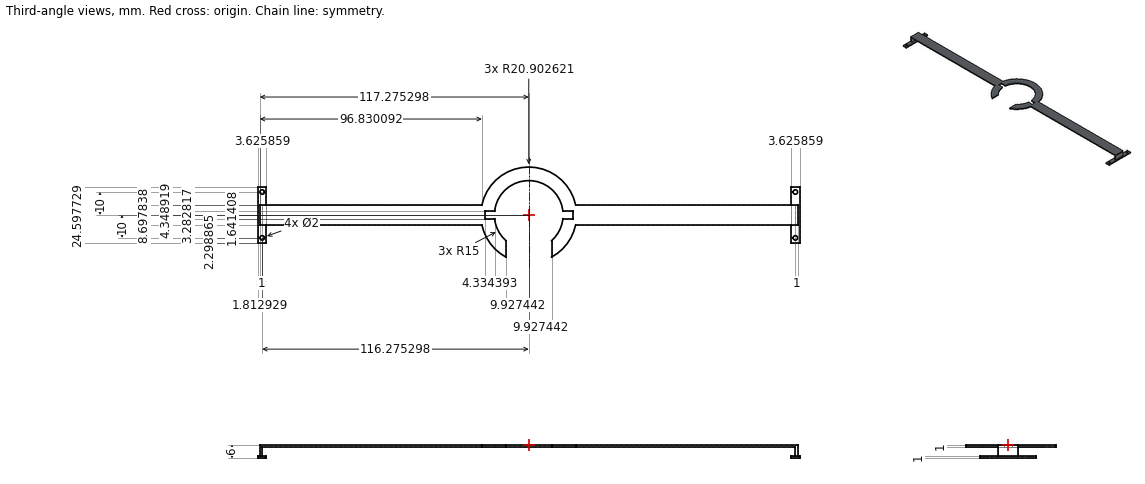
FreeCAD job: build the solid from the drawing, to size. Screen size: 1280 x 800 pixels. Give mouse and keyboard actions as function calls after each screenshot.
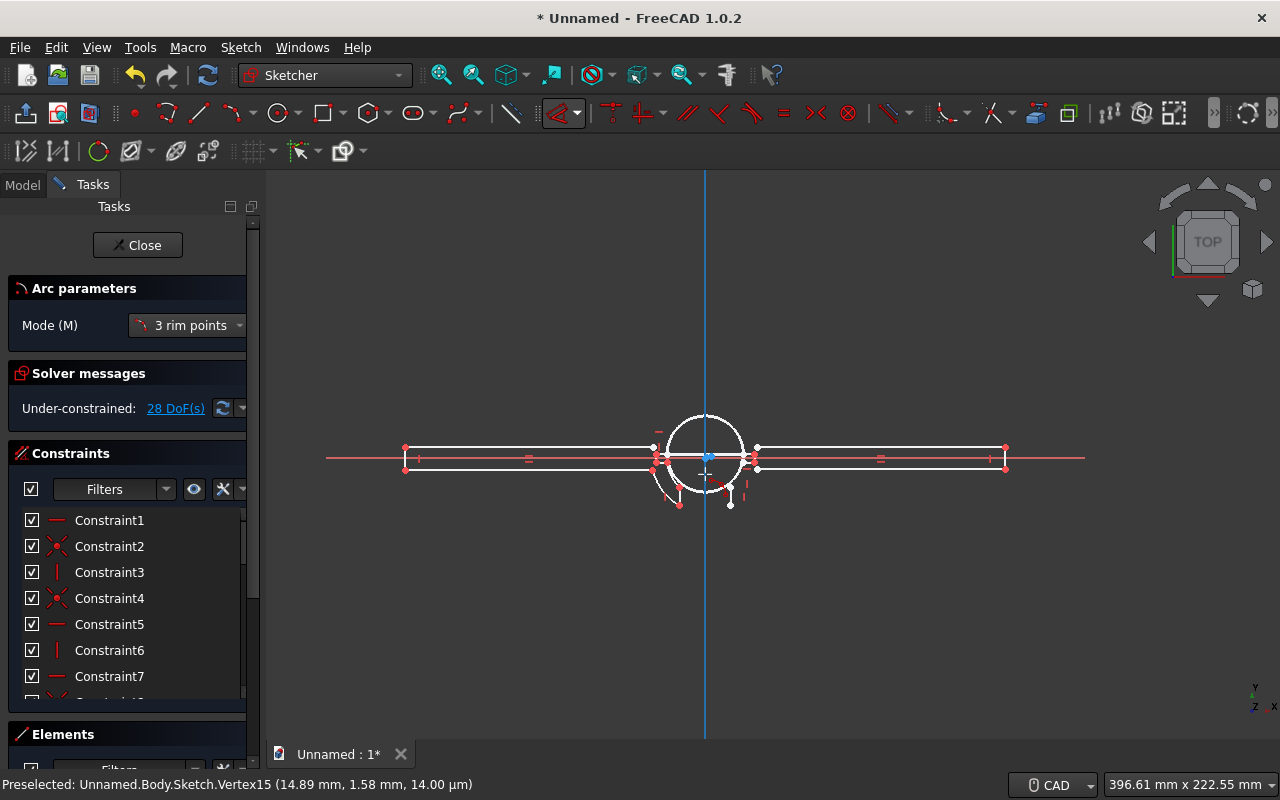
click(726, 426)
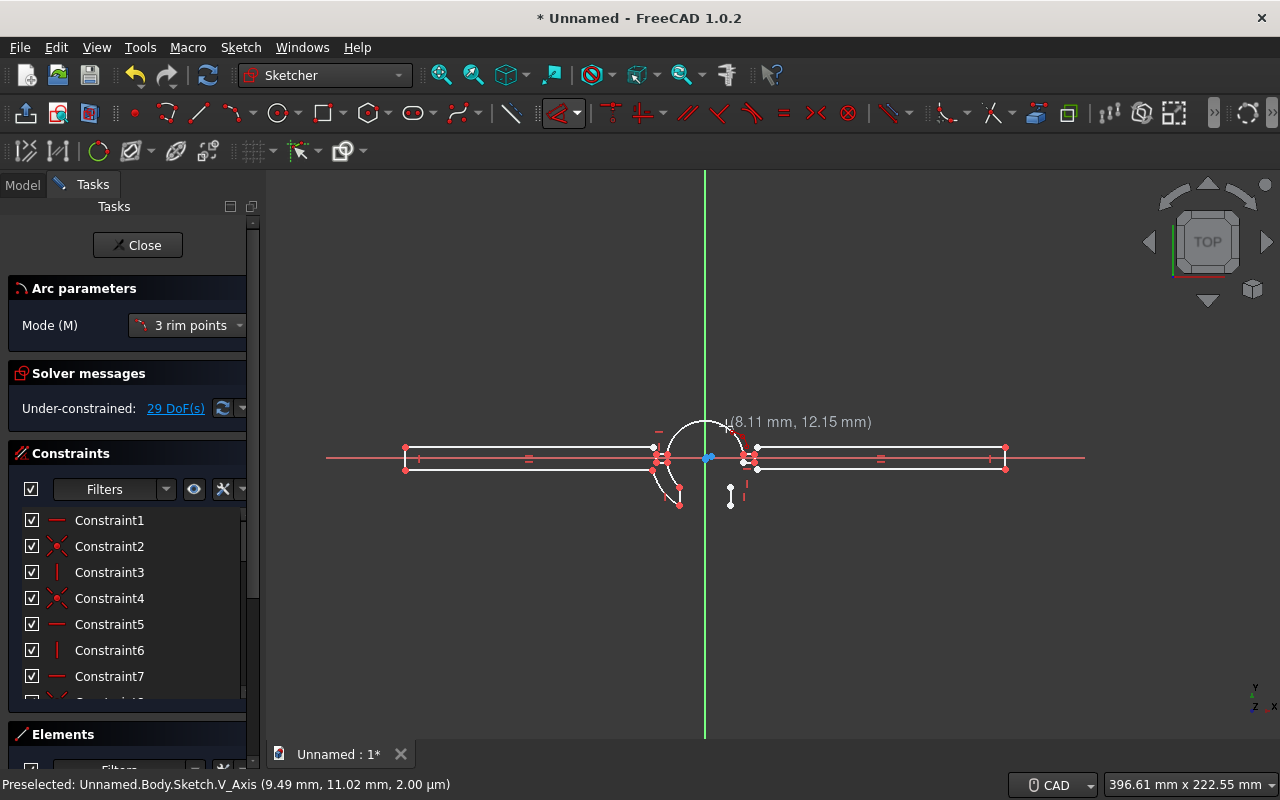
scroll(743, 462, up, 7)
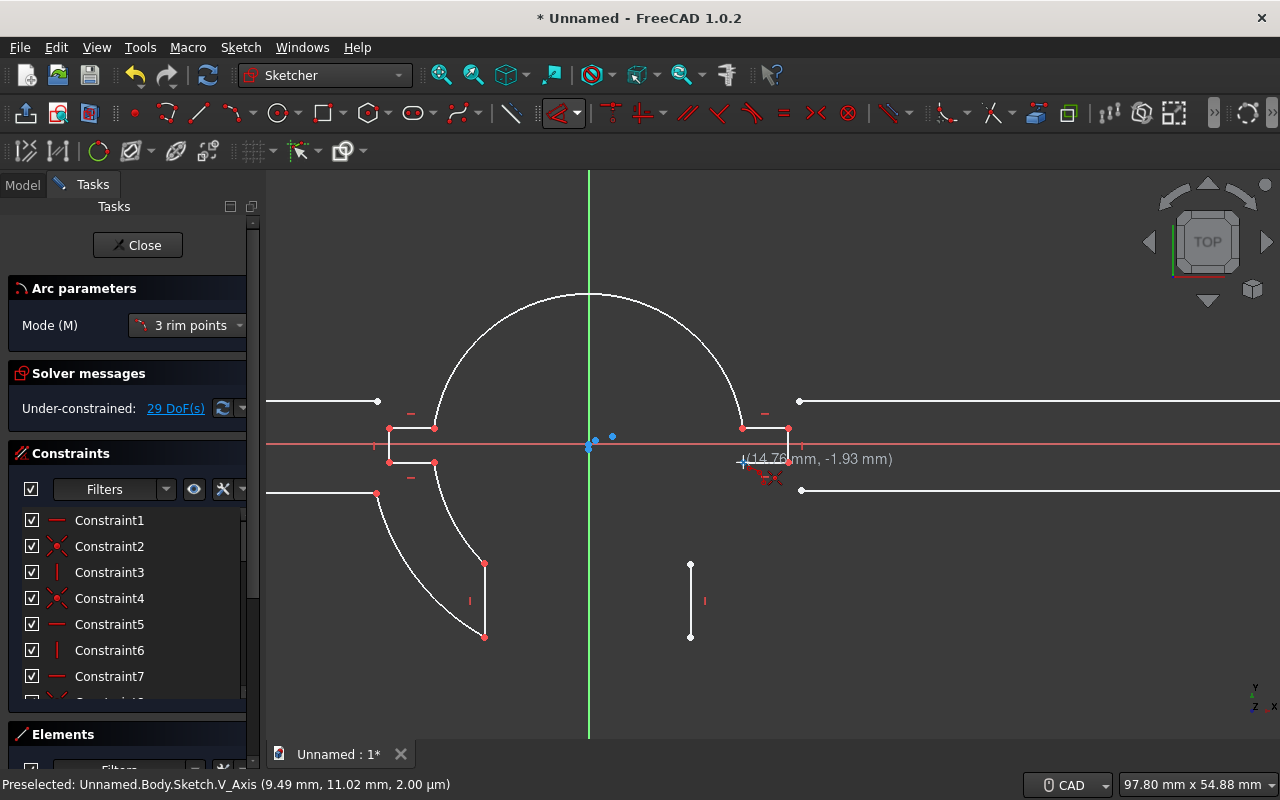
click(744, 463)
click(691, 565)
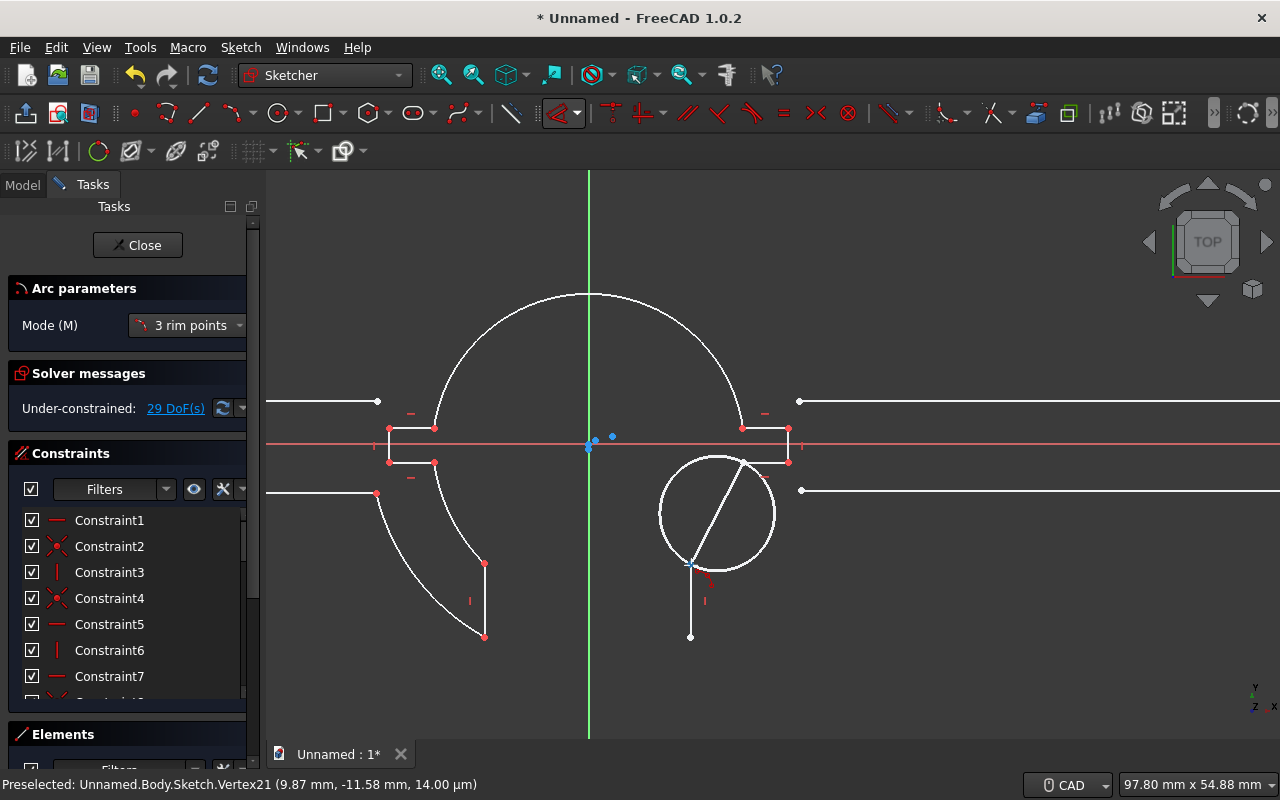
scroll(727, 516, up, 3)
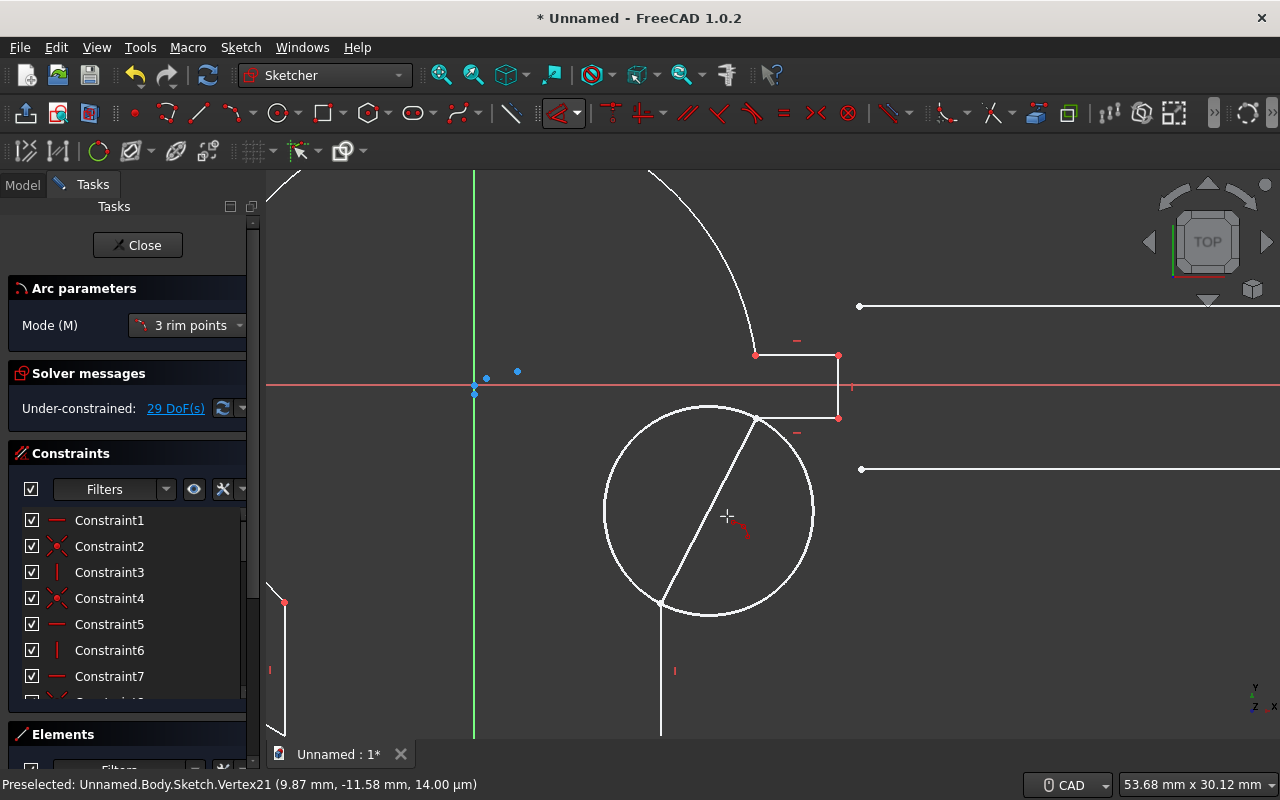
click(726, 516)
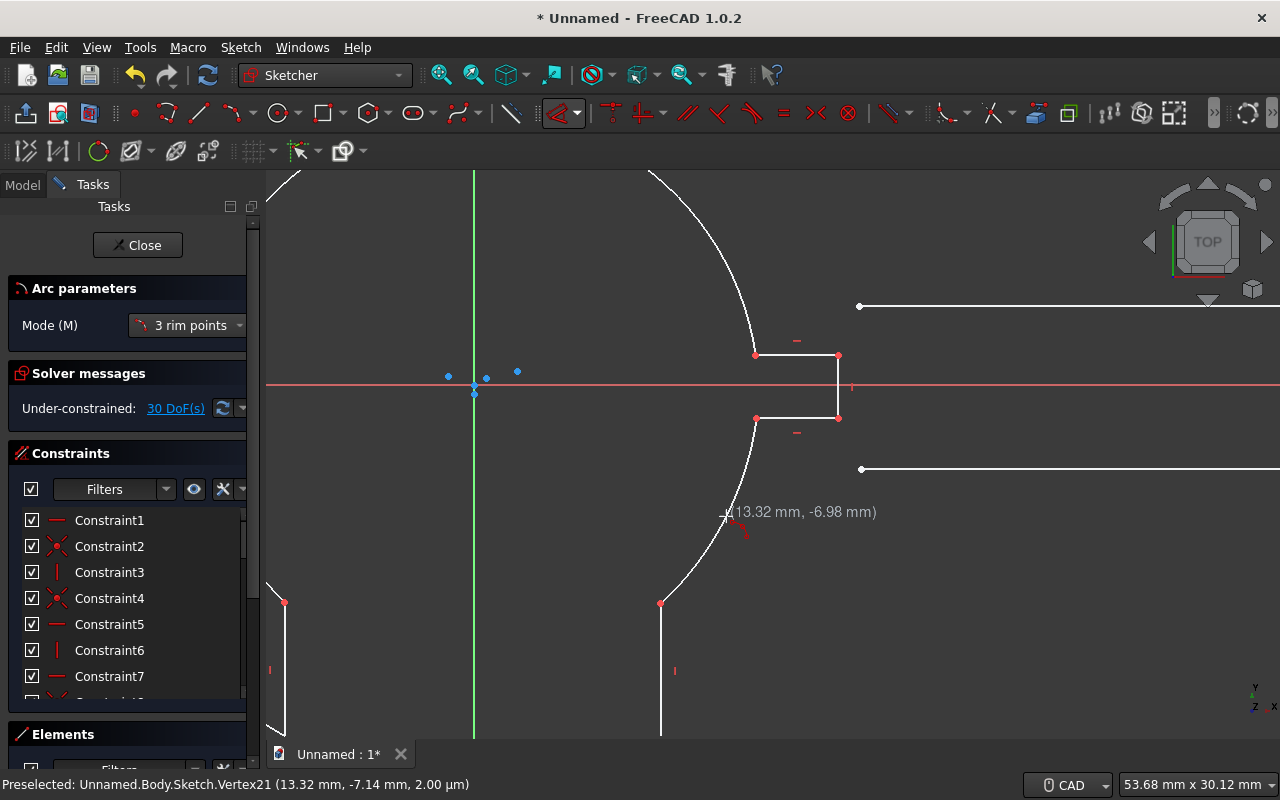
scroll(741, 469, down, 10)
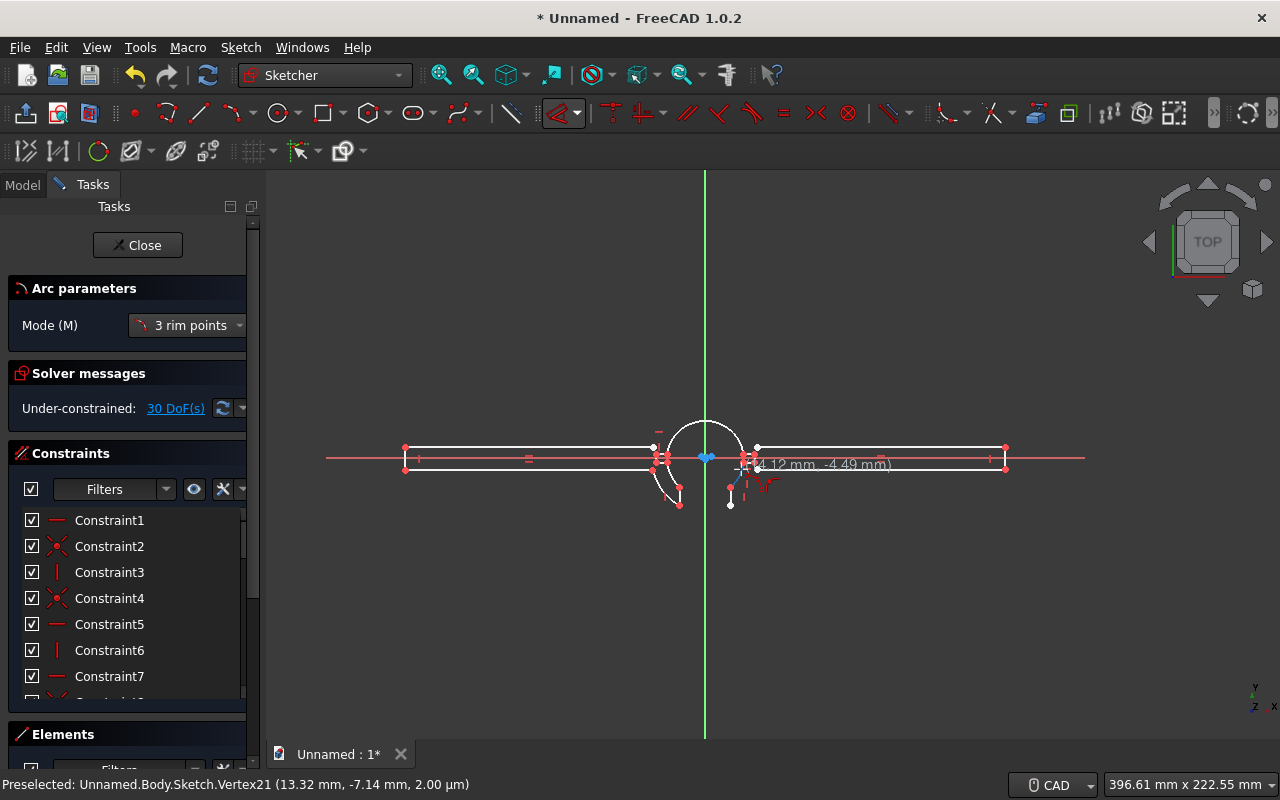
scroll(731, 505, up, 3)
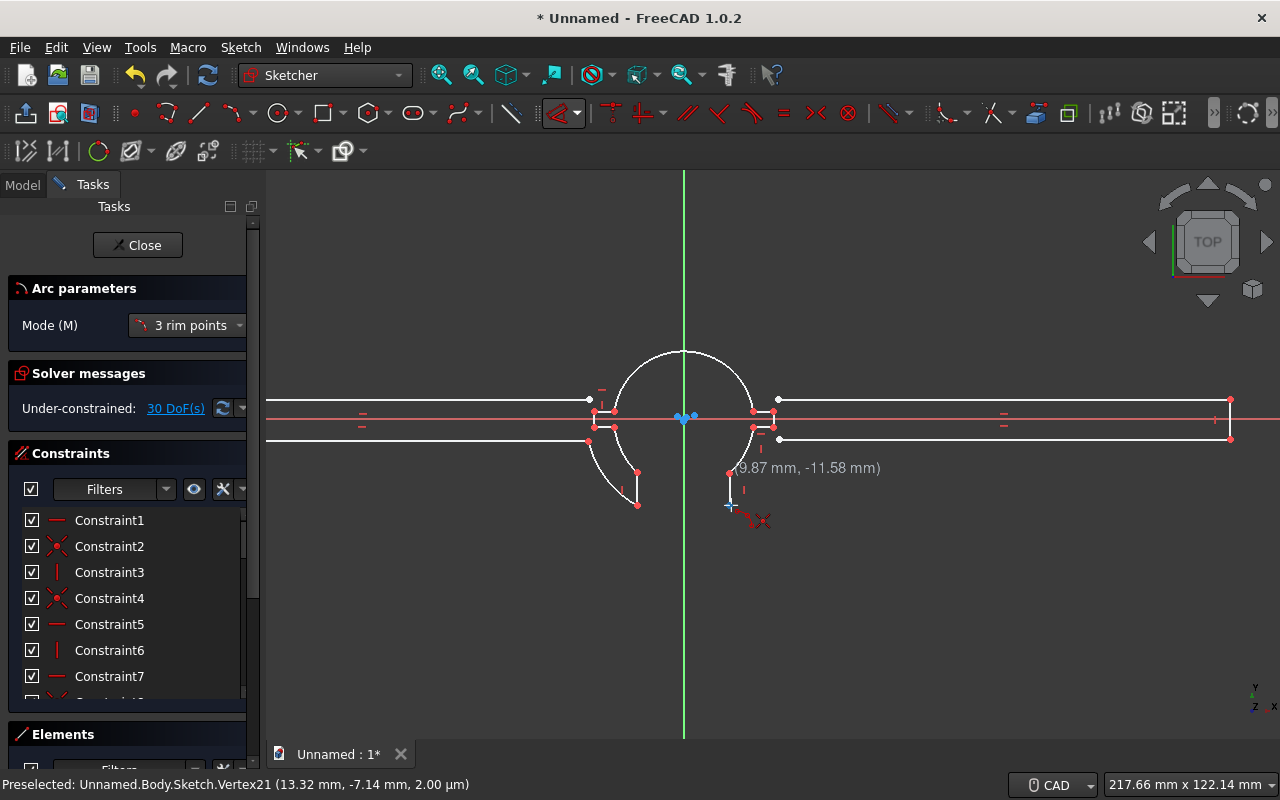
click(730, 506)
click(779, 440)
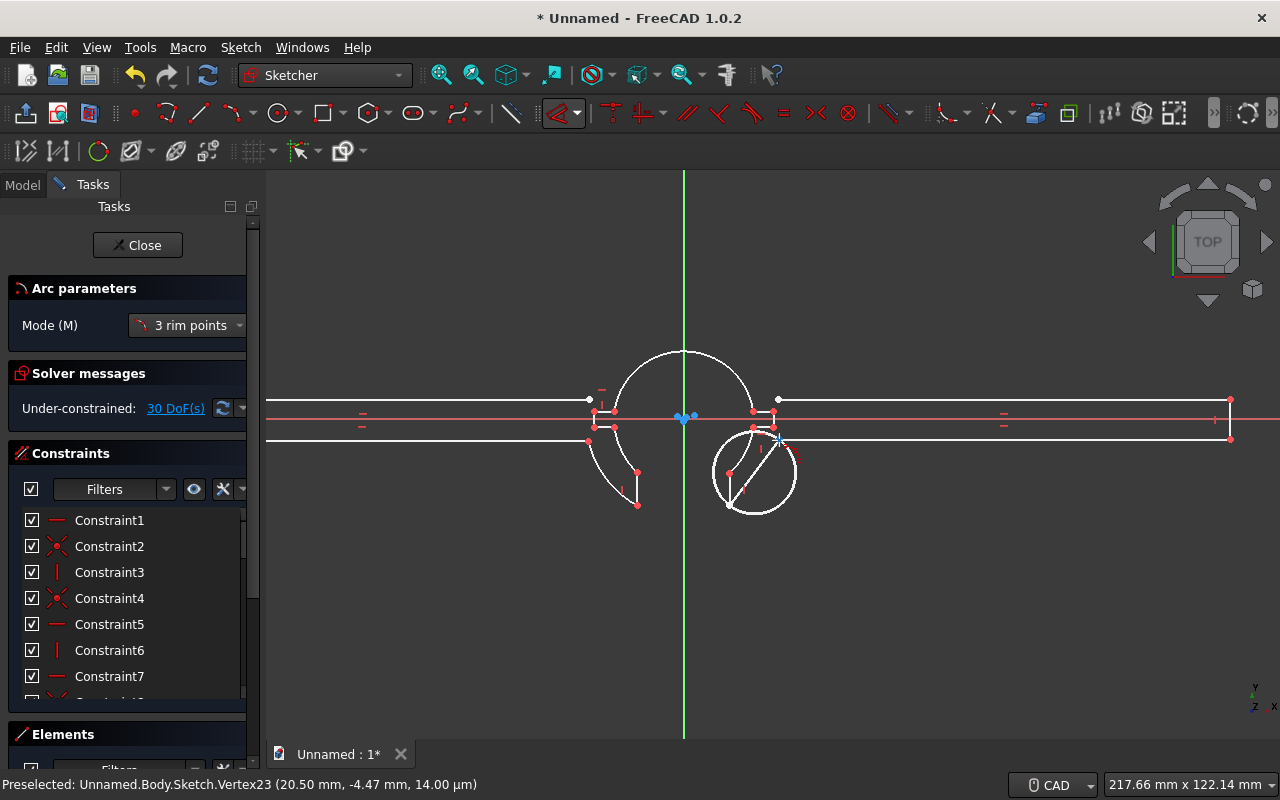
scroll(762, 477, up, 3)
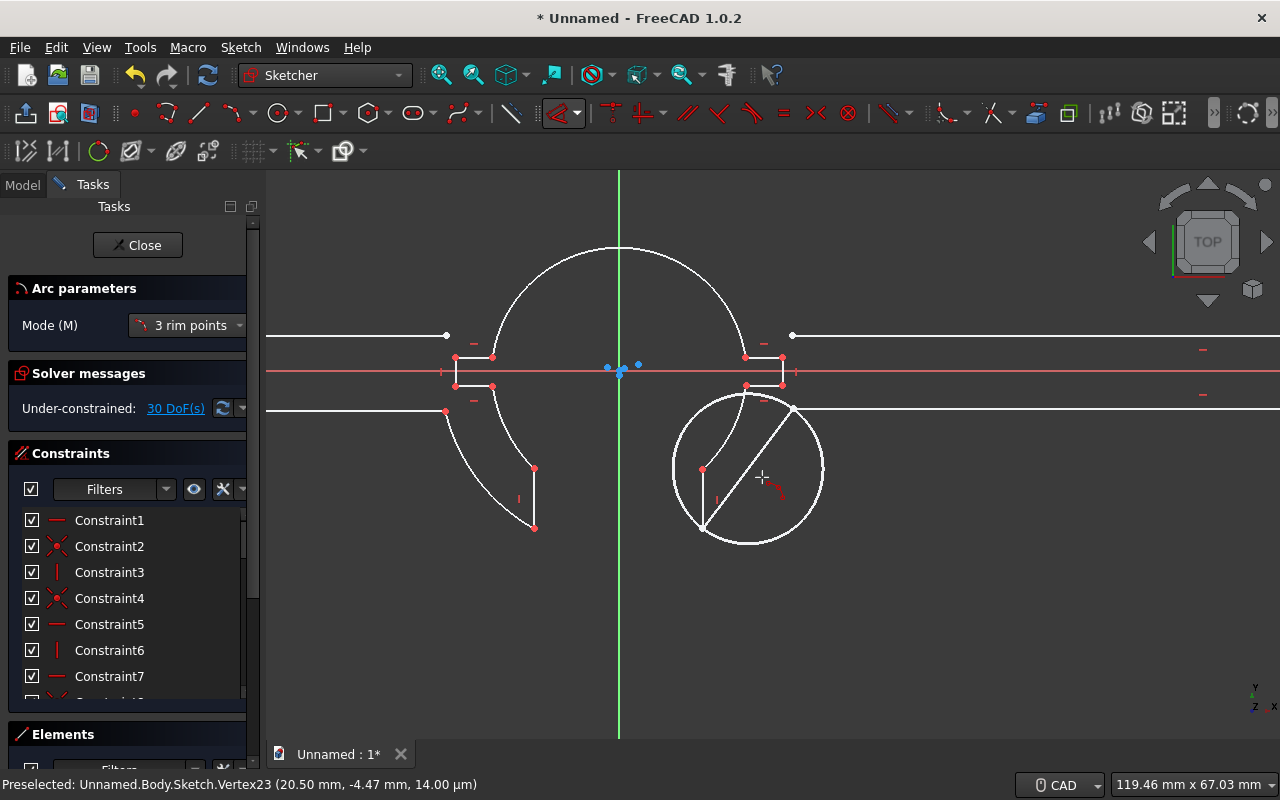
click(761, 477)